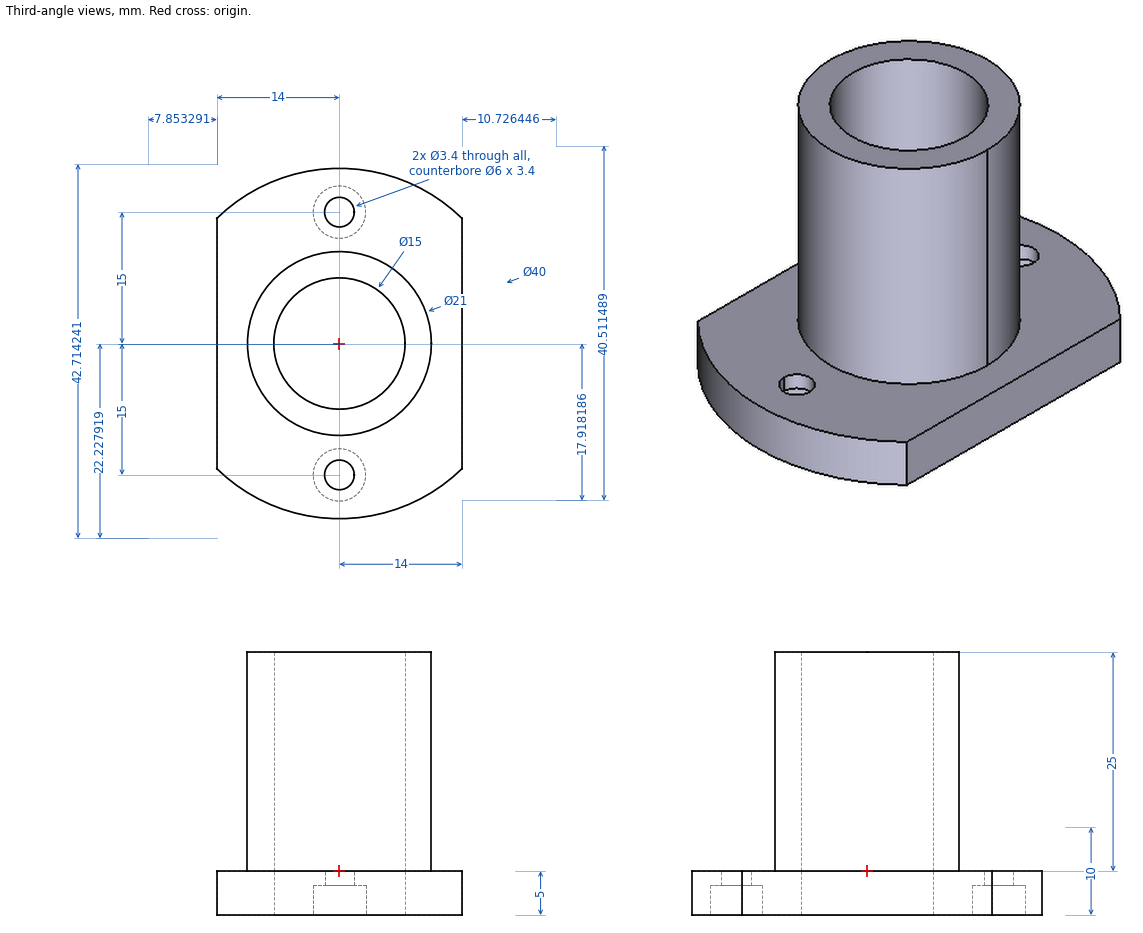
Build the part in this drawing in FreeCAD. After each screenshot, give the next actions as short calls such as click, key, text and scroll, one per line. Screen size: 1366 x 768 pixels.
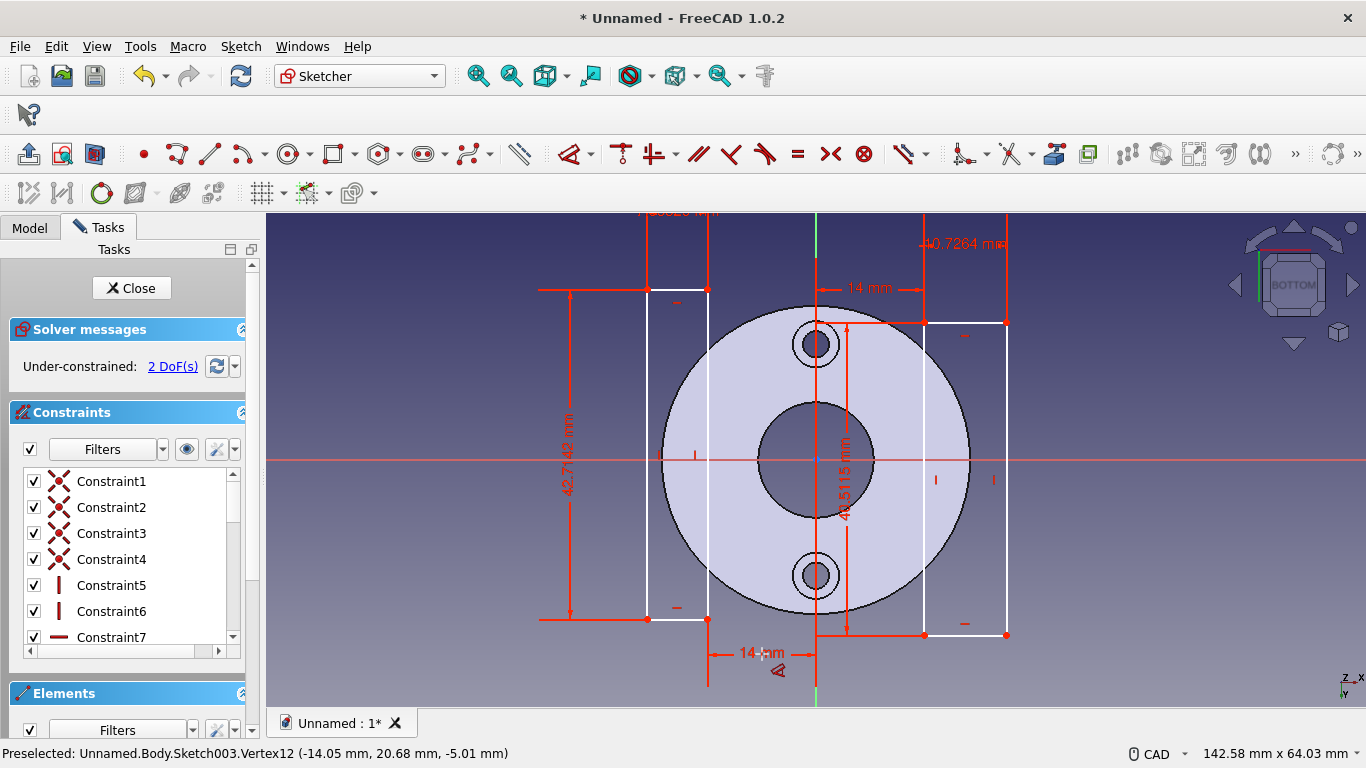
click(924, 323)
click(958, 392)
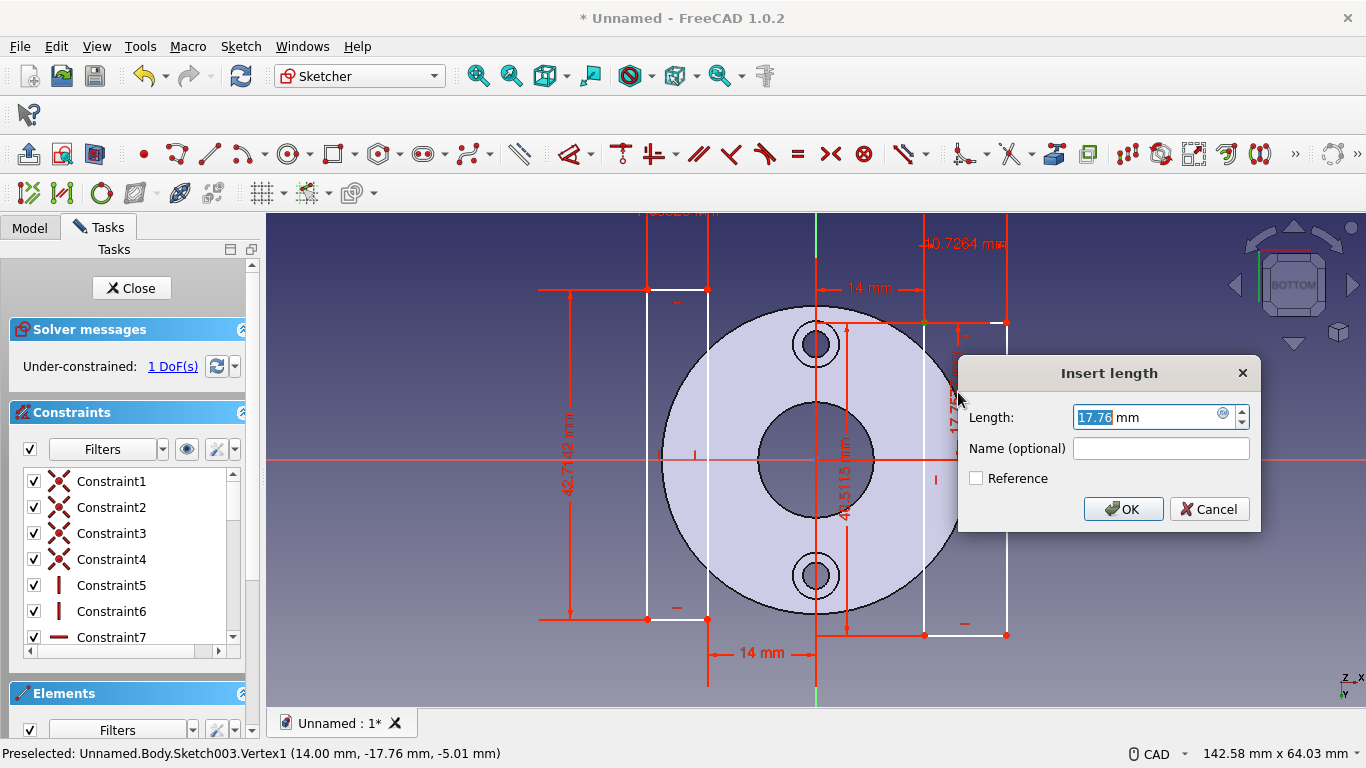
text(17.918186)
key(Return)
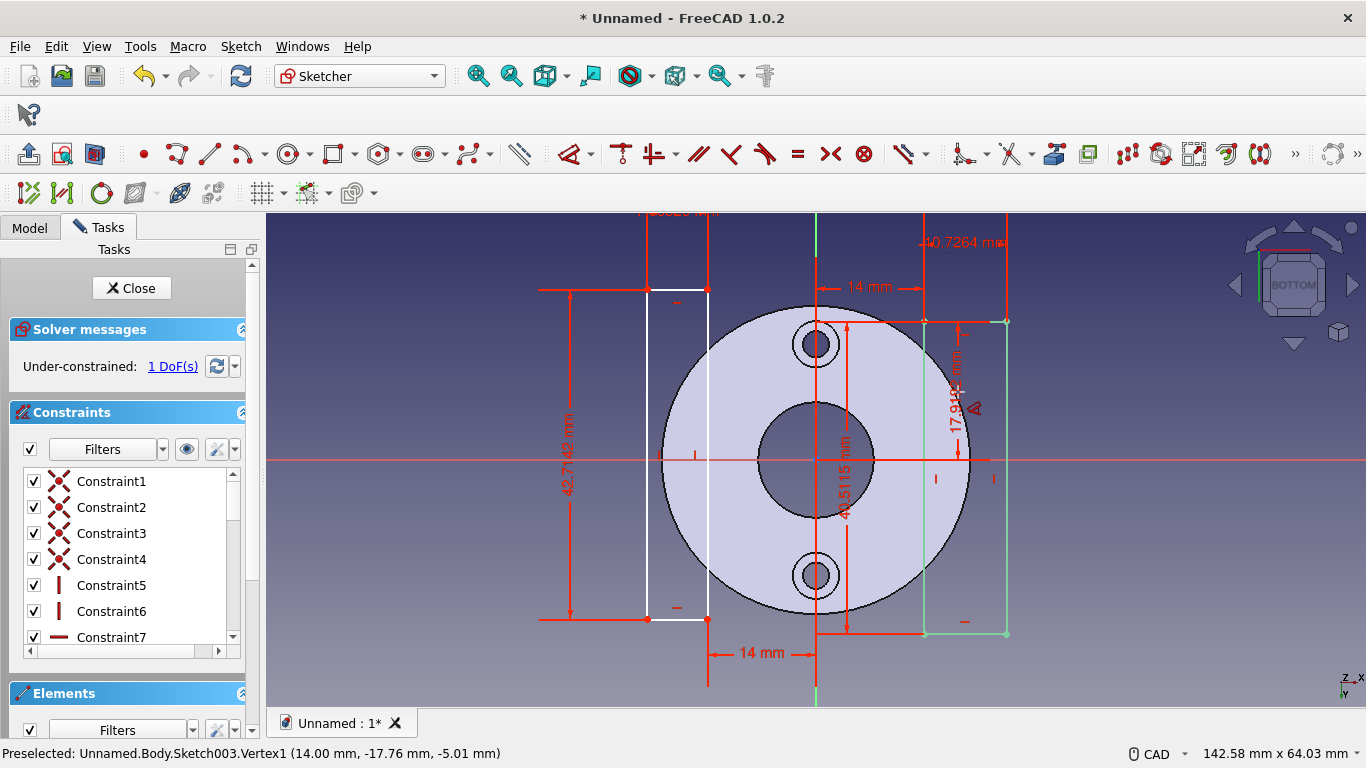
click(647, 290)
click(613, 375)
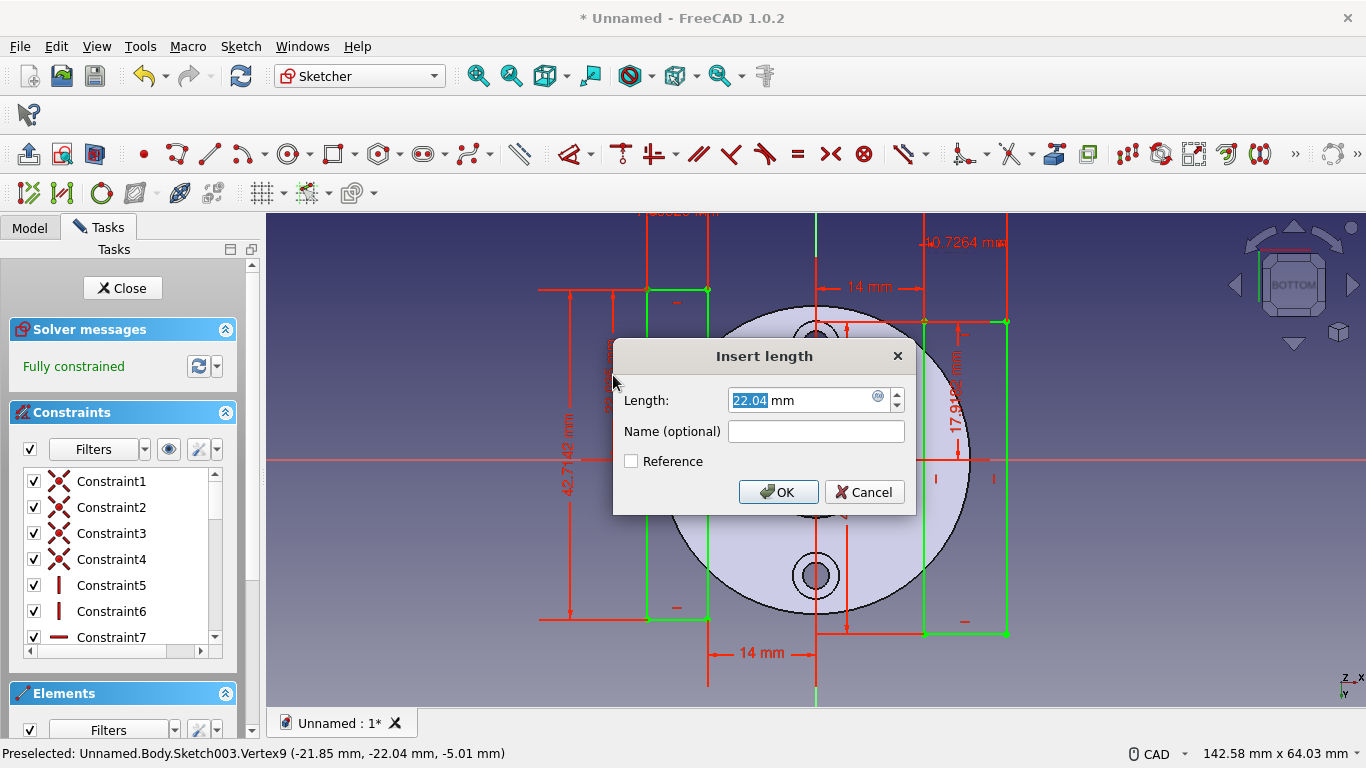
text(22.227919)
key(Return)
key(Escape)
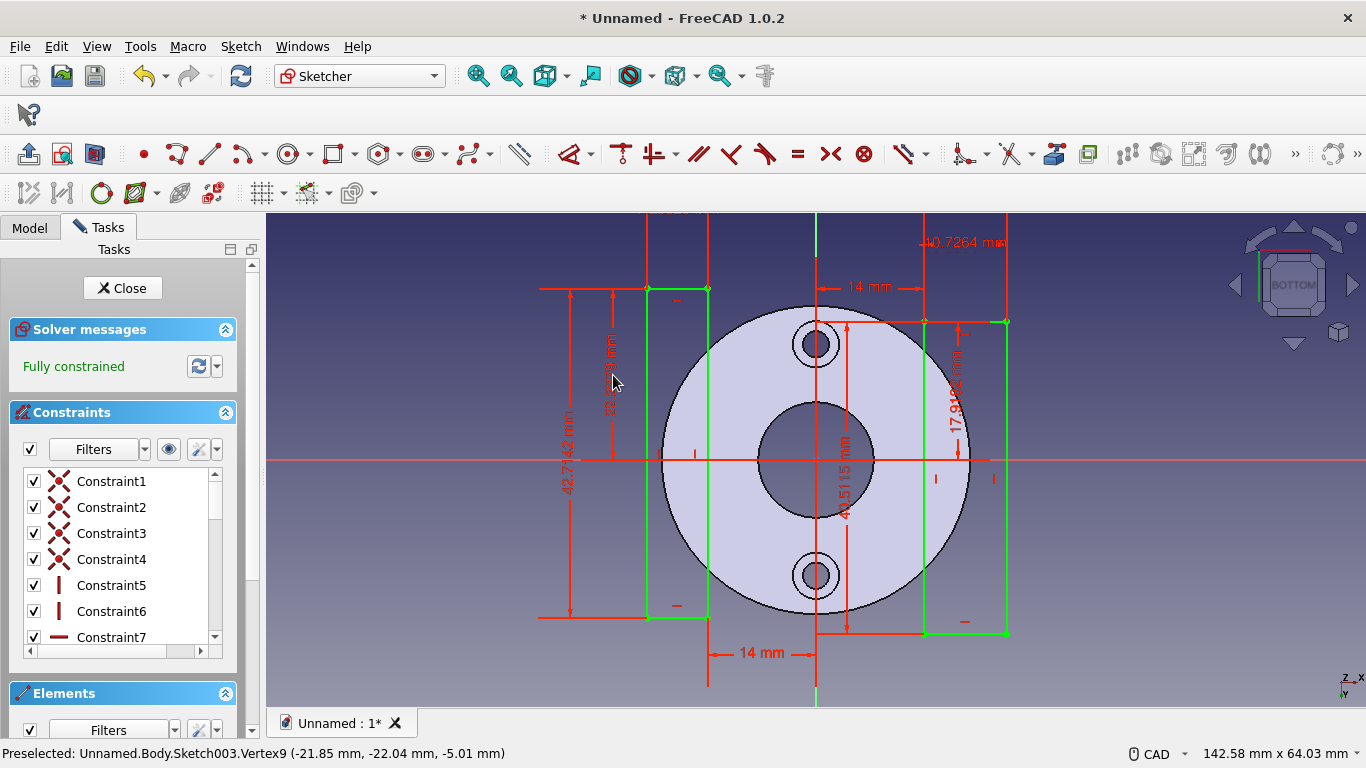
click(123, 288)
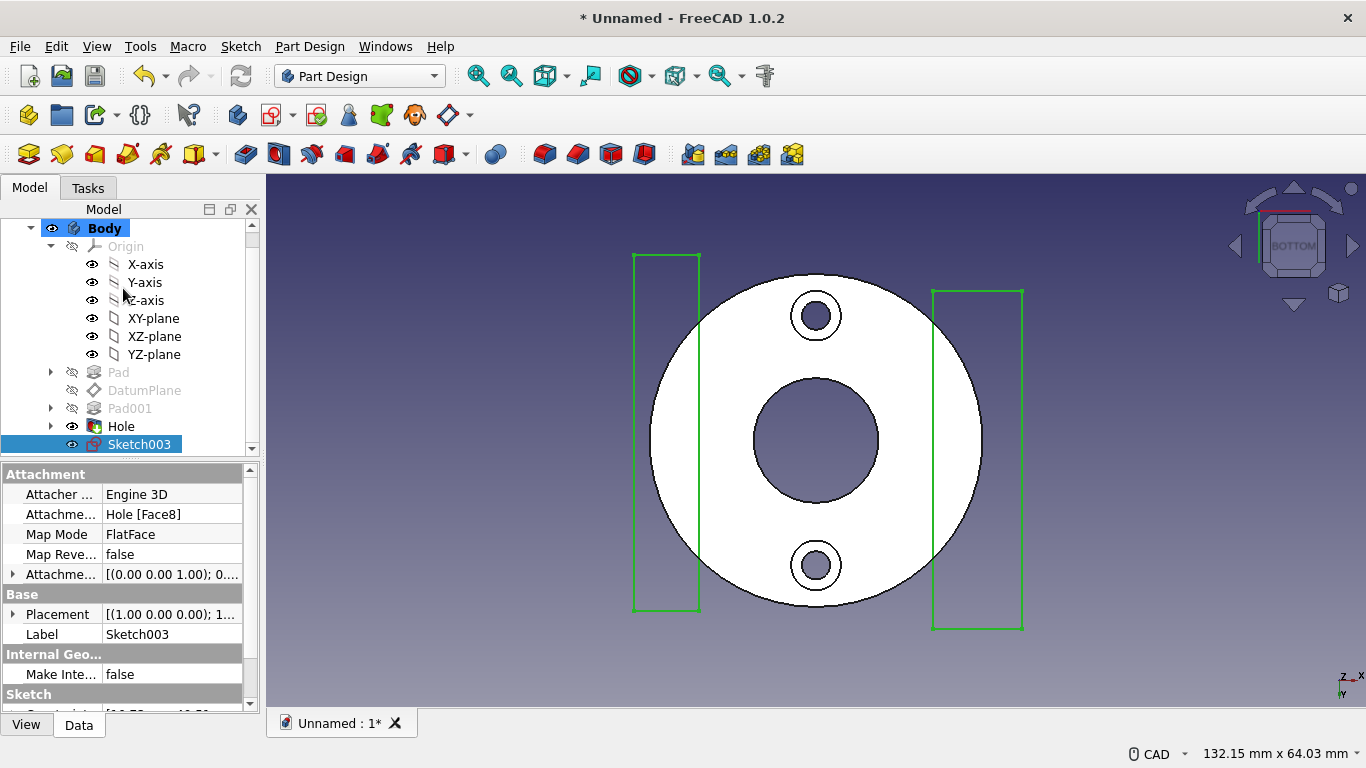
click(246, 154)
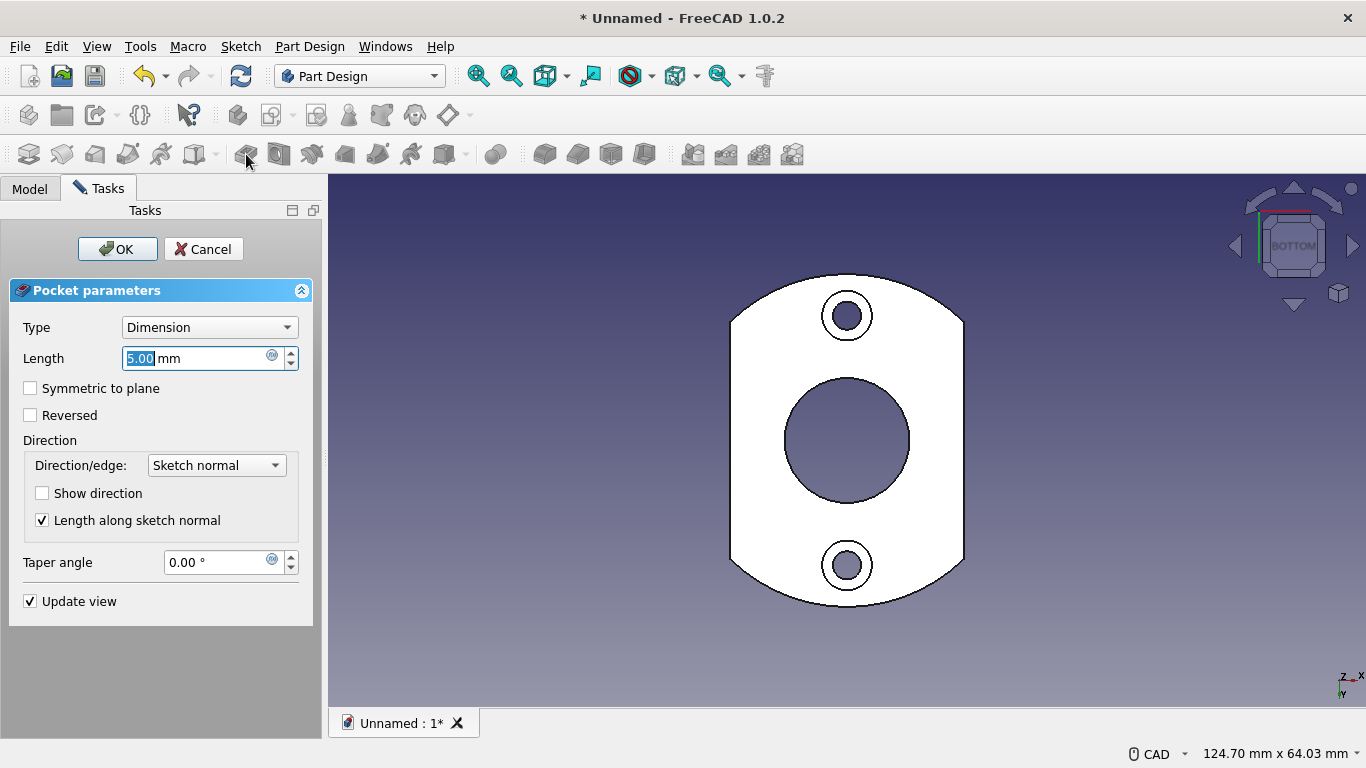
text(10)
key(Tab)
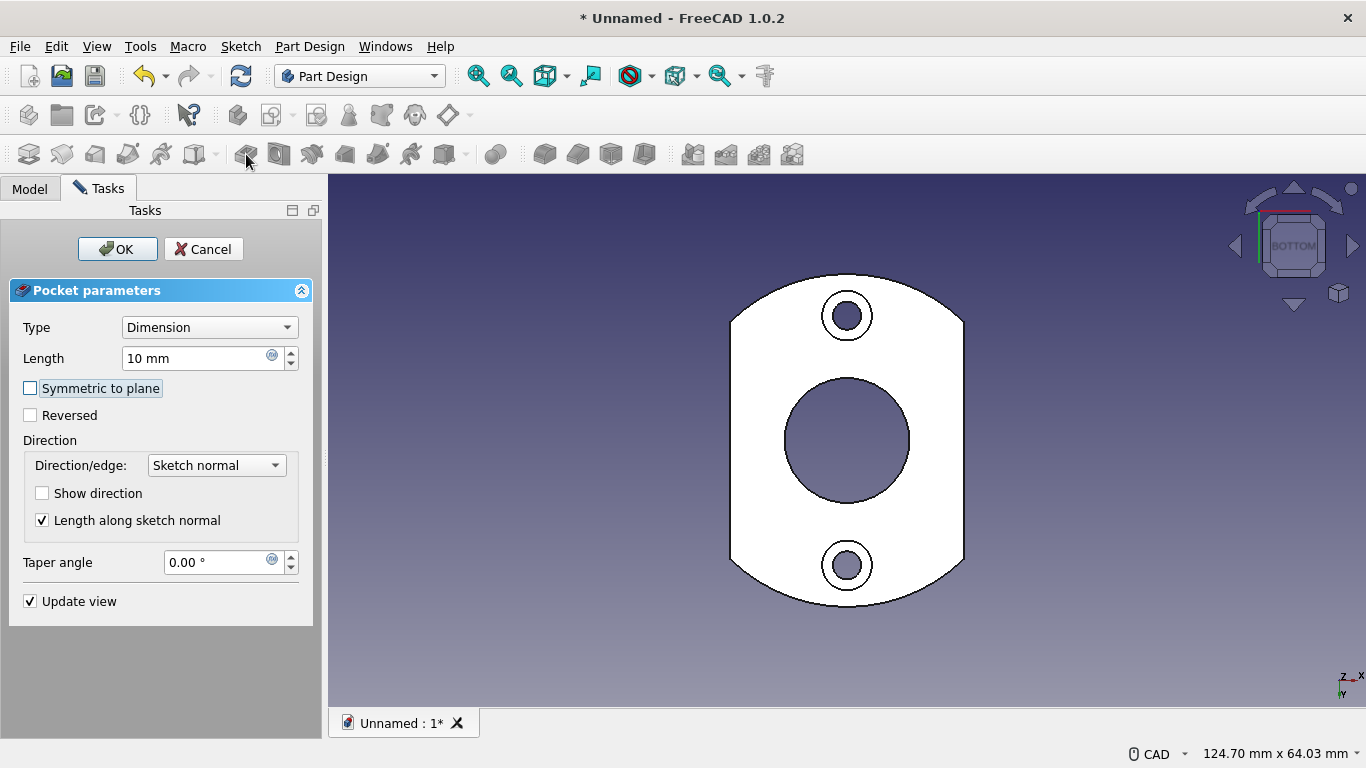
click(118, 249)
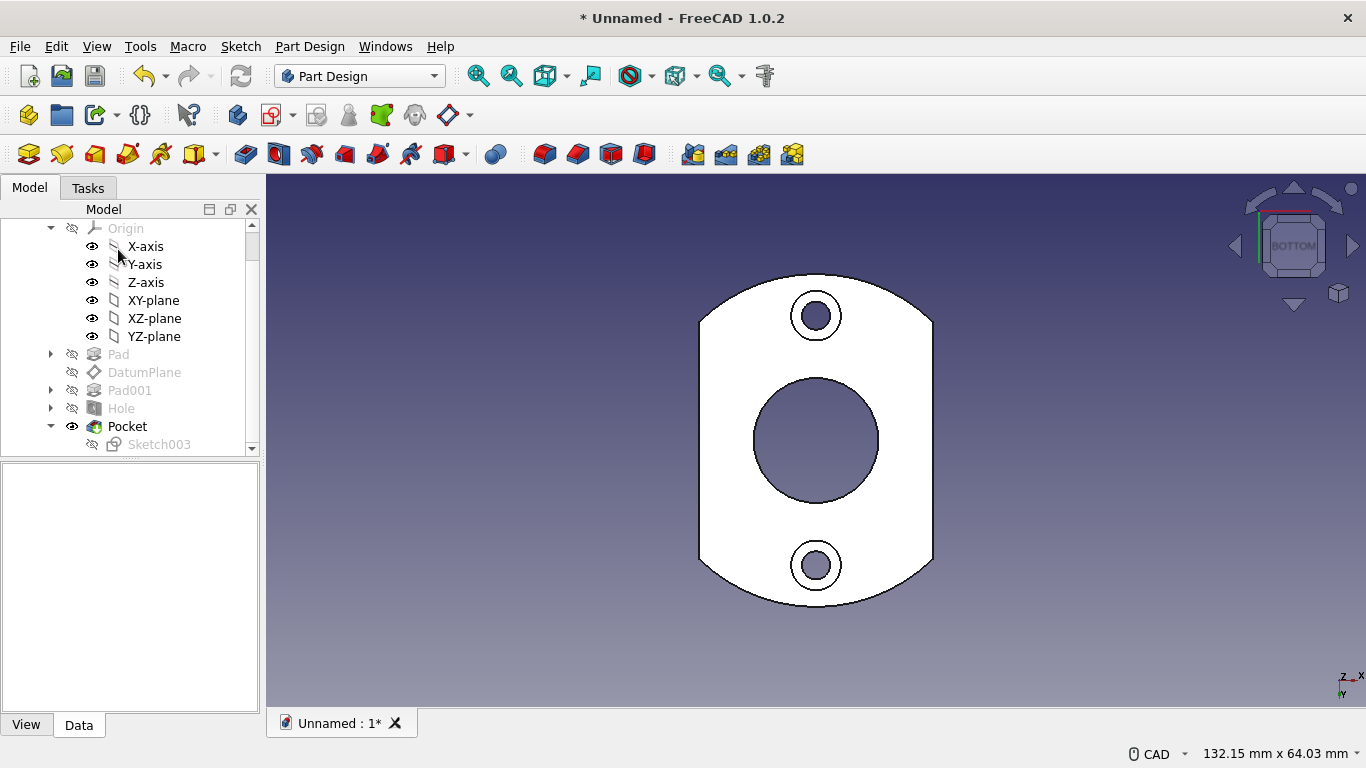
key(0)